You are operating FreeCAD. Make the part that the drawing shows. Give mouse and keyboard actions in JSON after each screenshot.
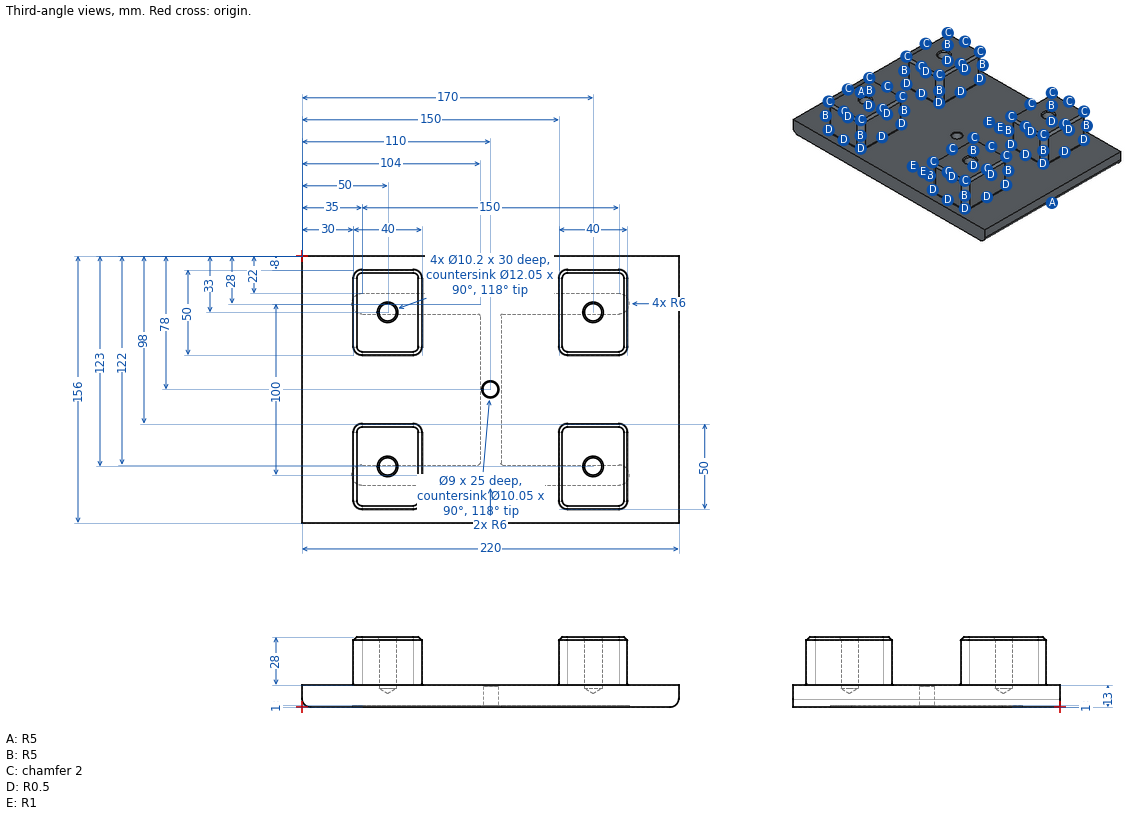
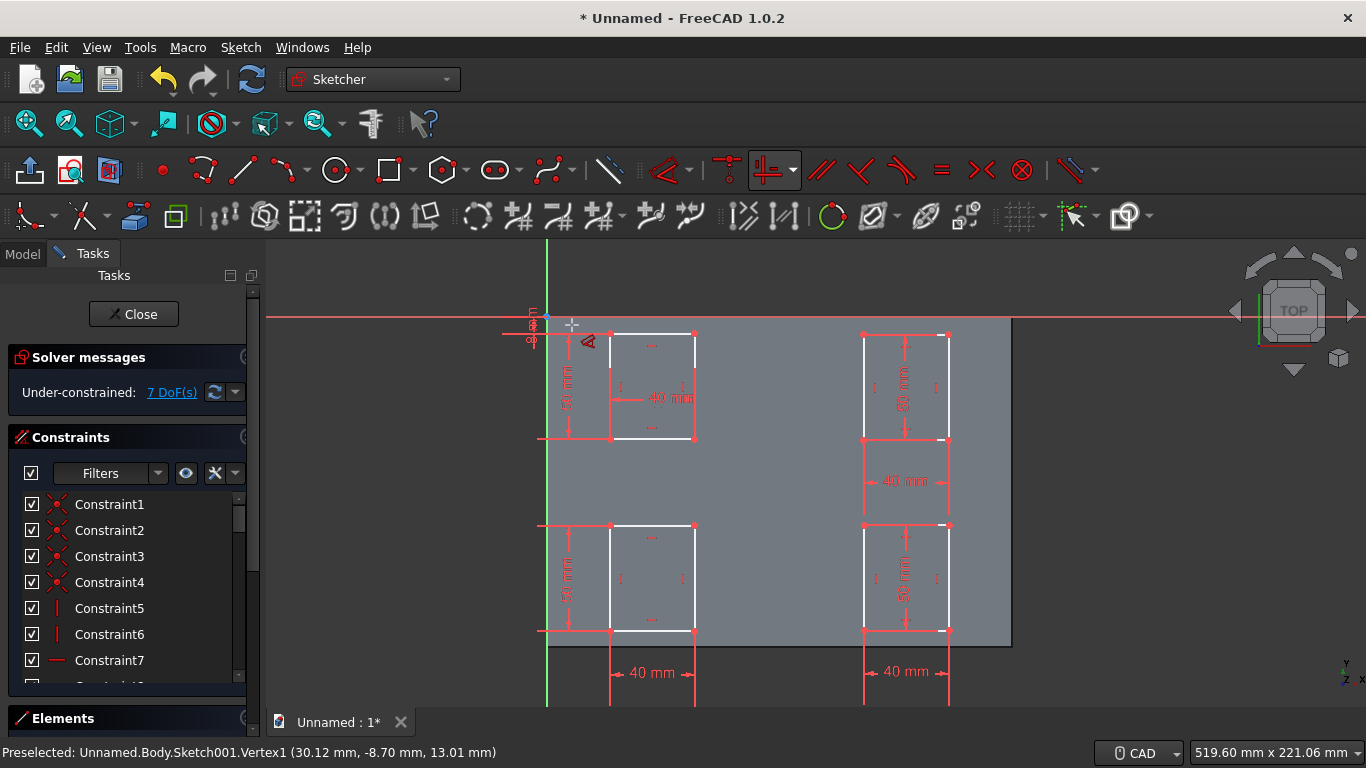
{"action": "scroll", "coordinate": [864, 335], "scroll_direction": "up", "scroll_amount": 5}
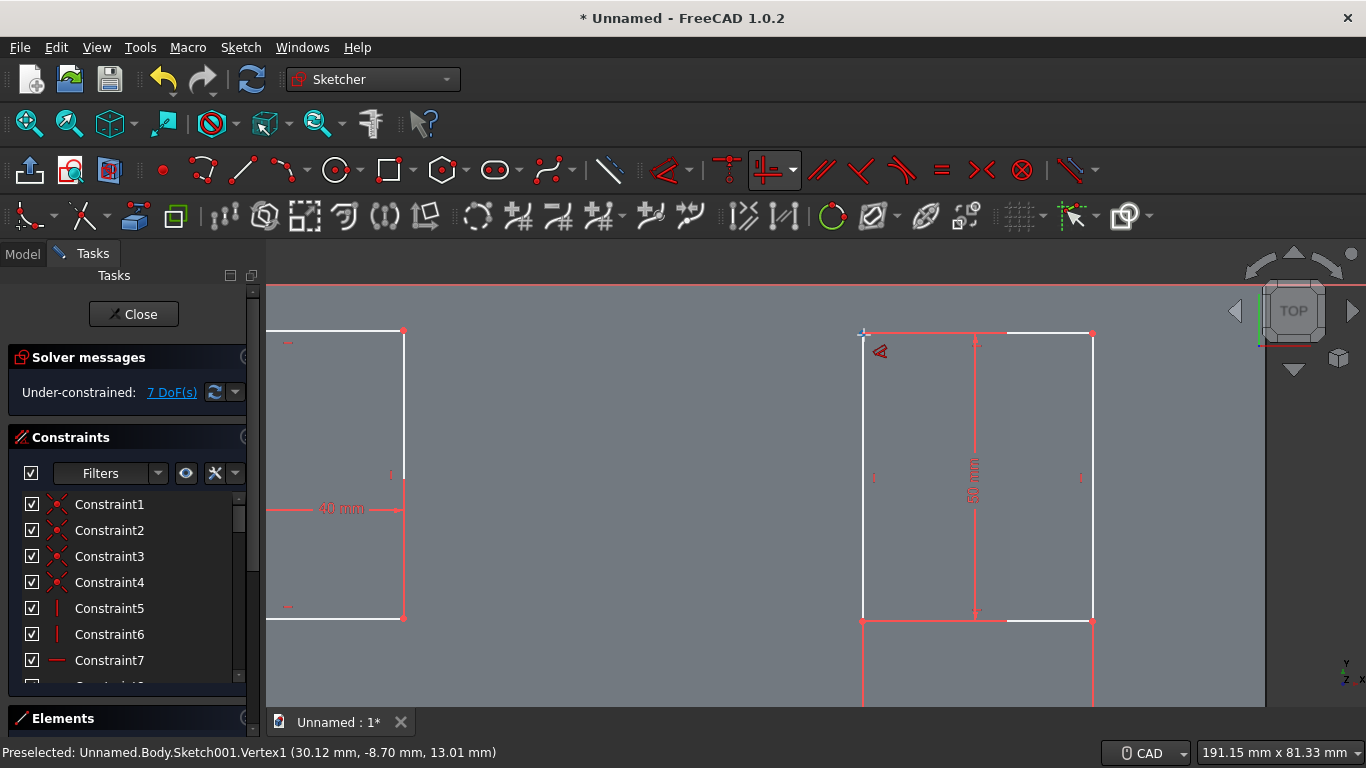
{"action": "left_click", "coordinate": [863, 333]}
{"action": "left_click", "coordinate": [897, 309]}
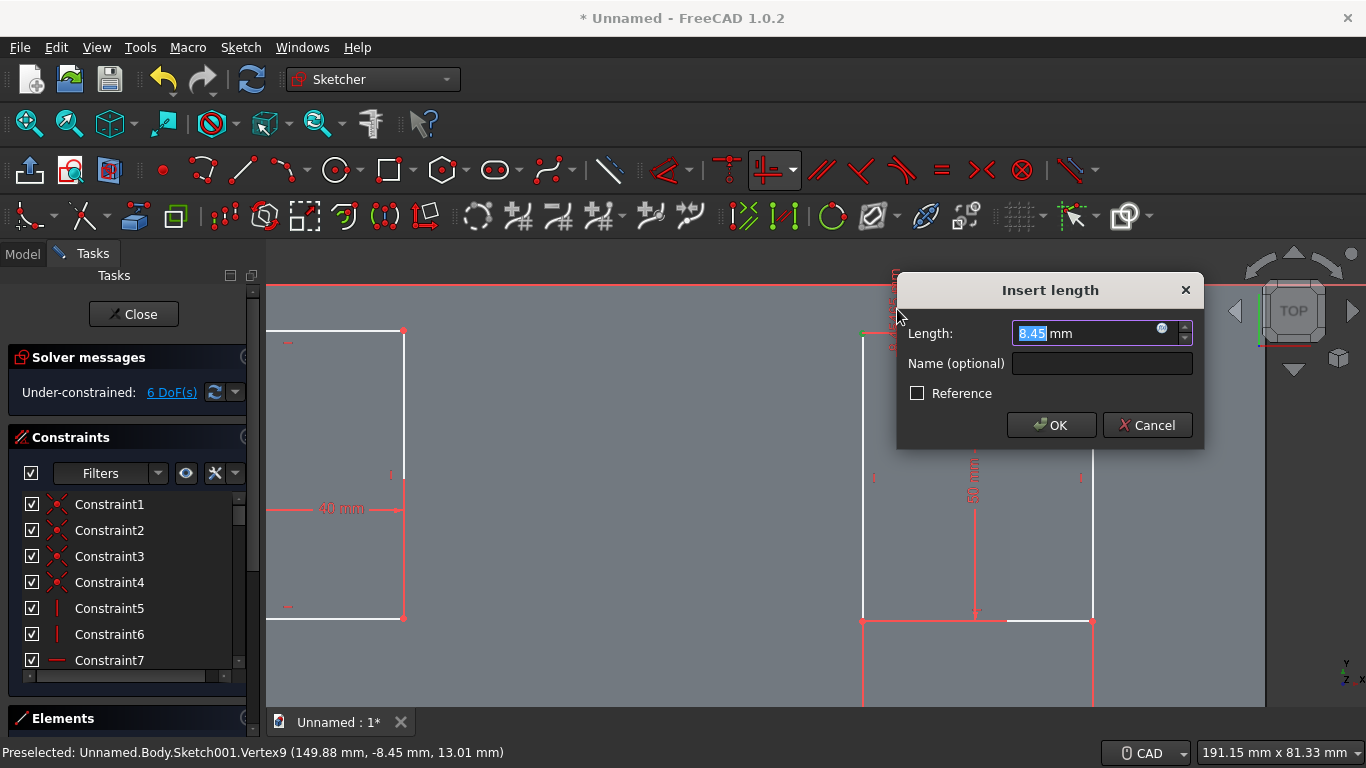
{"action": "type", "text": "8"}
{"action": "key", "text": "Return"}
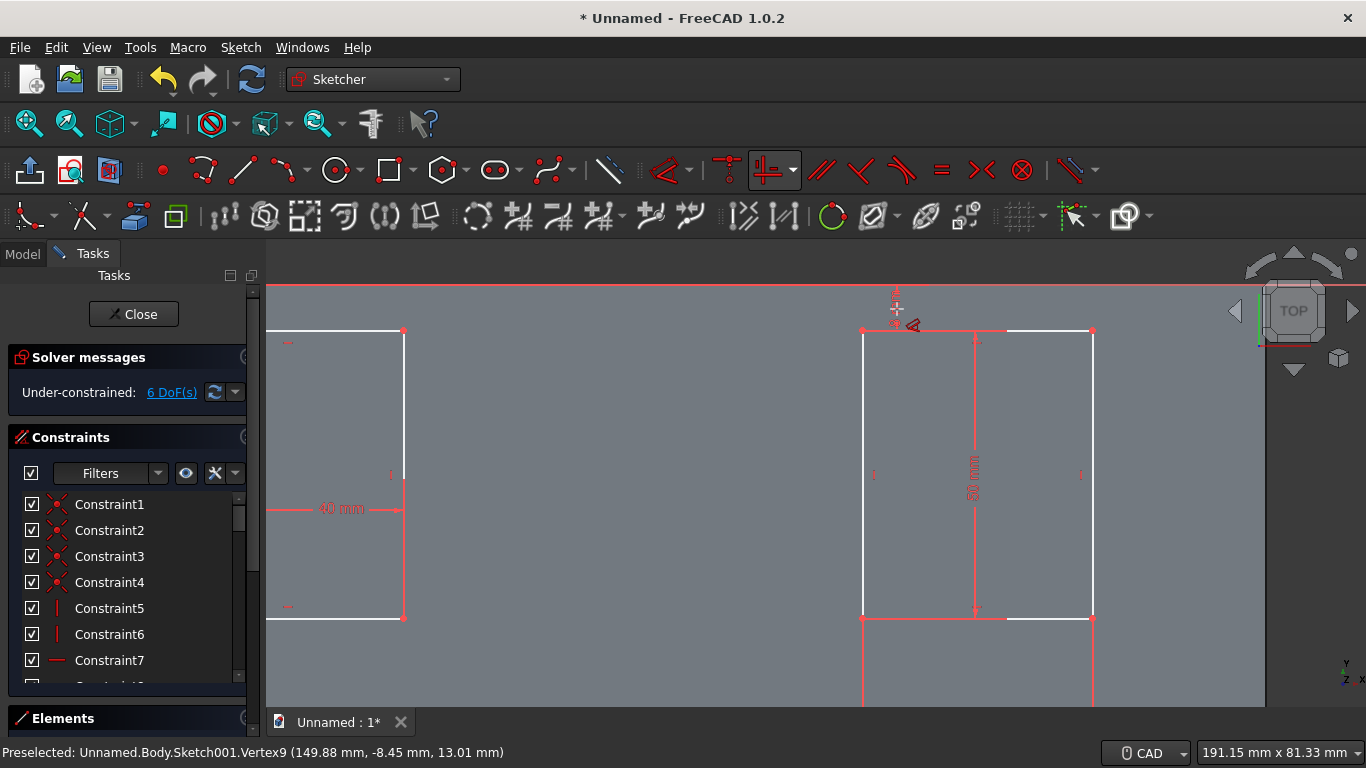
{"action": "scroll", "coordinate": [864, 335], "scroll_direction": "down", "scroll_amount": 5}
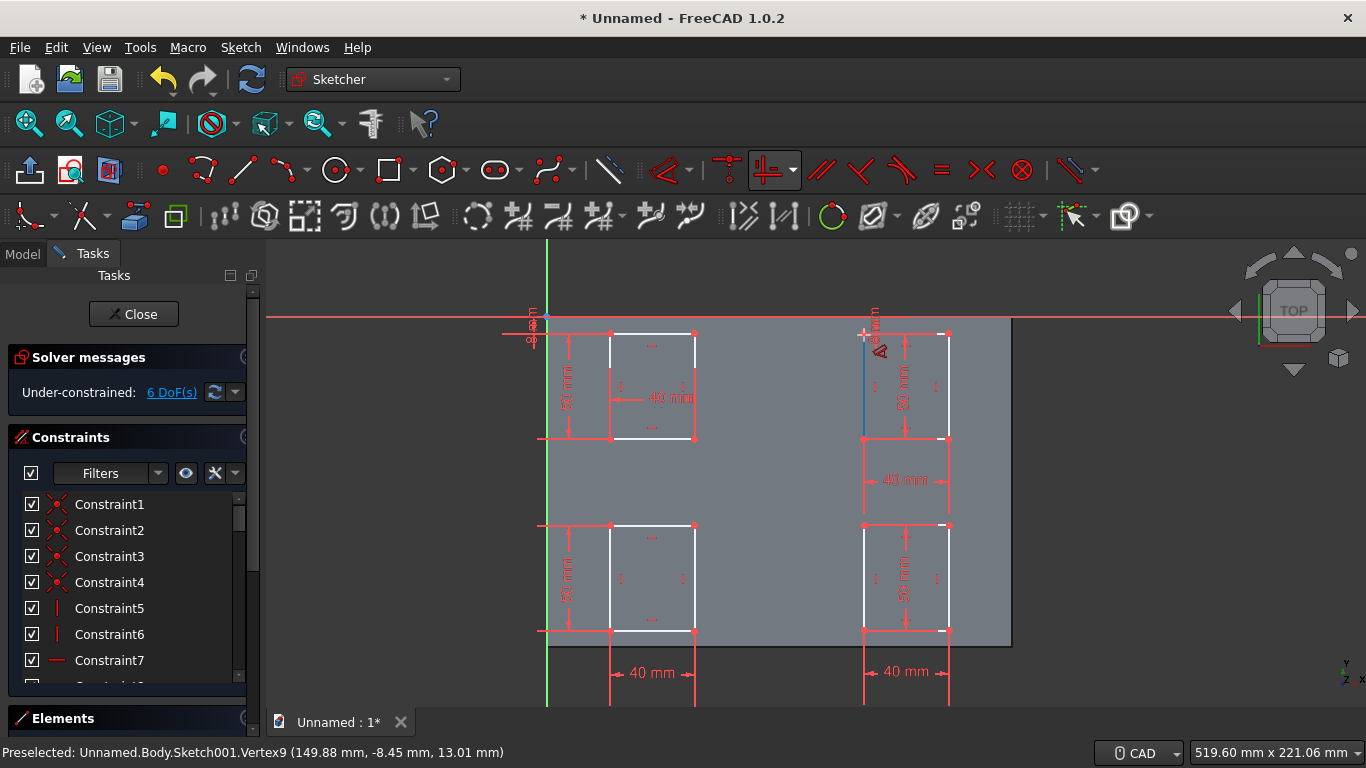
{"action": "left_click", "coordinate": [610, 334]}
{"action": "left_click", "coordinate": [578, 283]}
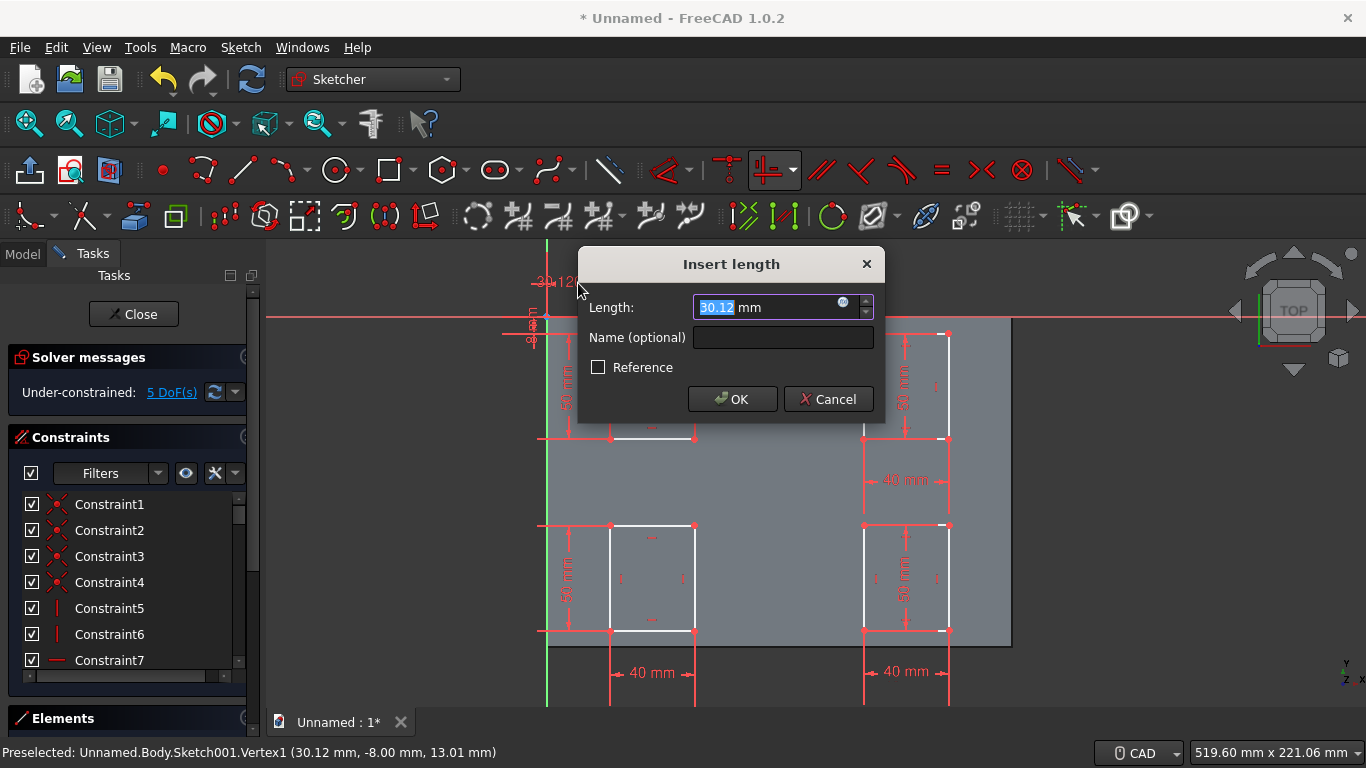
{"action": "type", "text": "30"}
{"action": "key", "text": "Return"}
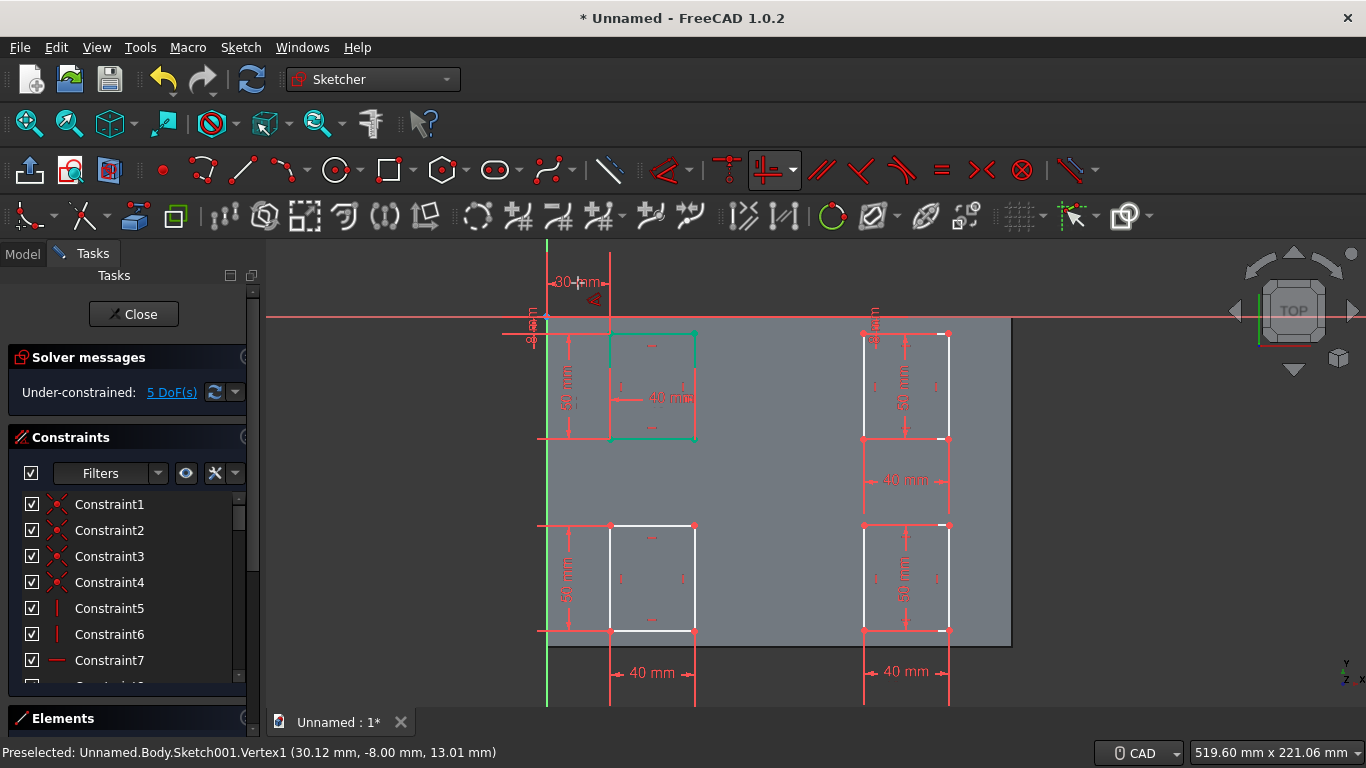
{"action": "left_click", "coordinate": [864, 525]}
{"action": "left_click", "coordinate": [513, 421]}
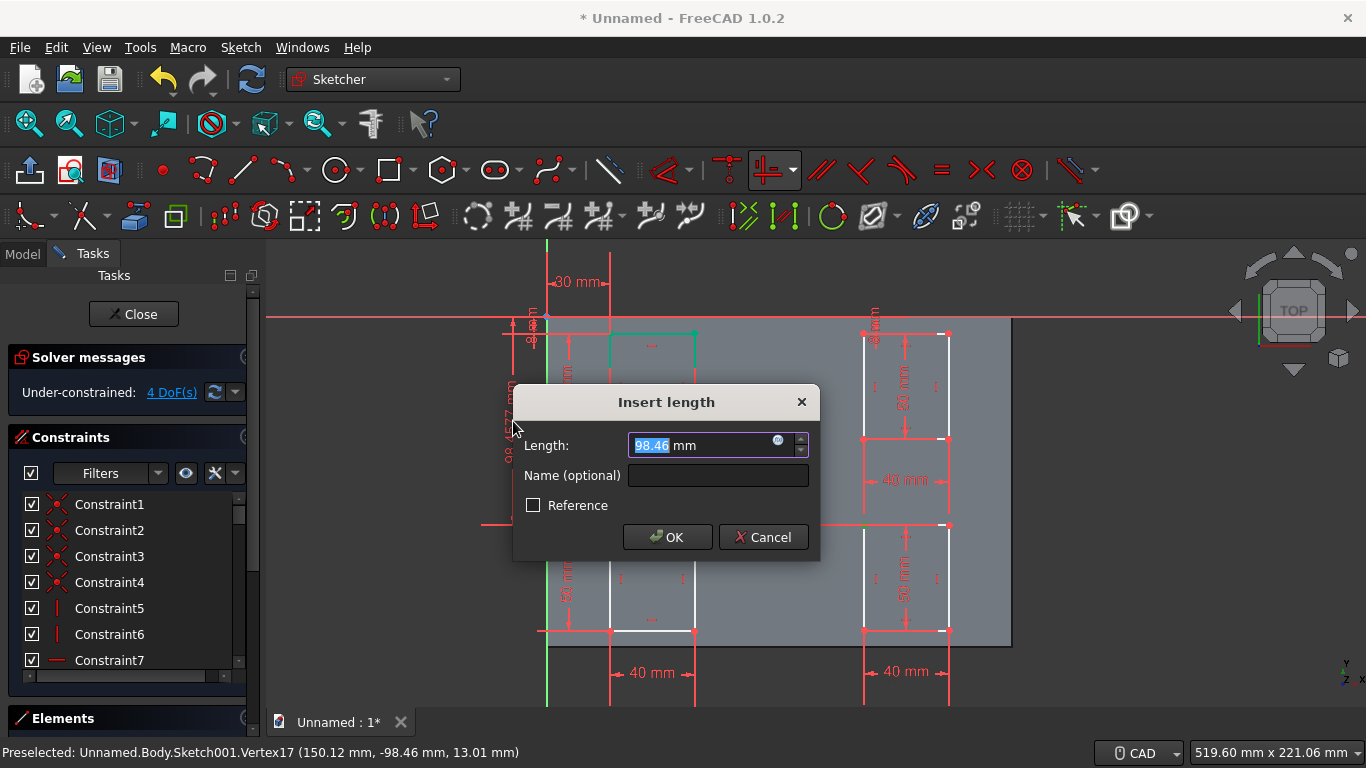
{"action": "type", "text": "98"}
{"action": "key", "text": "Return"}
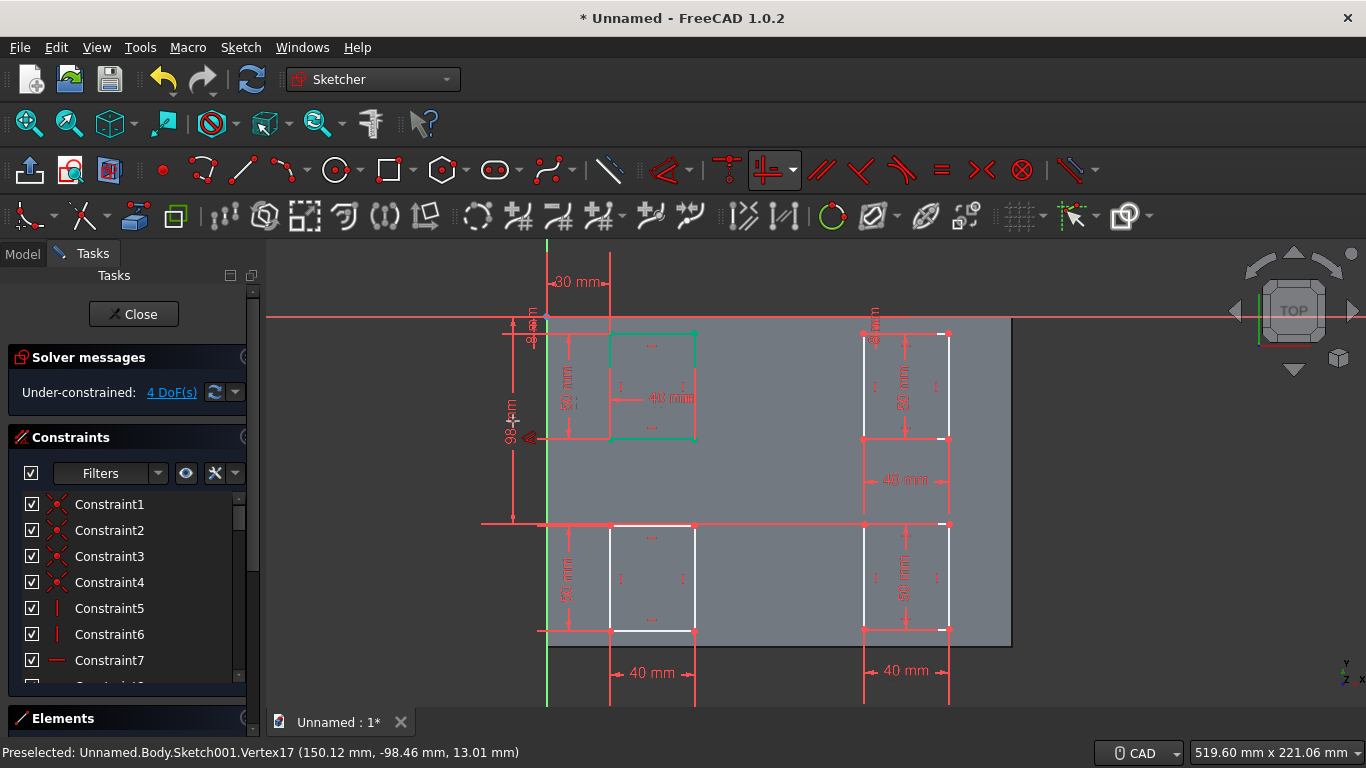
{"action": "left_click", "coordinate": [610, 526]}
{"action": "left_click", "coordinate": [578, 608]}